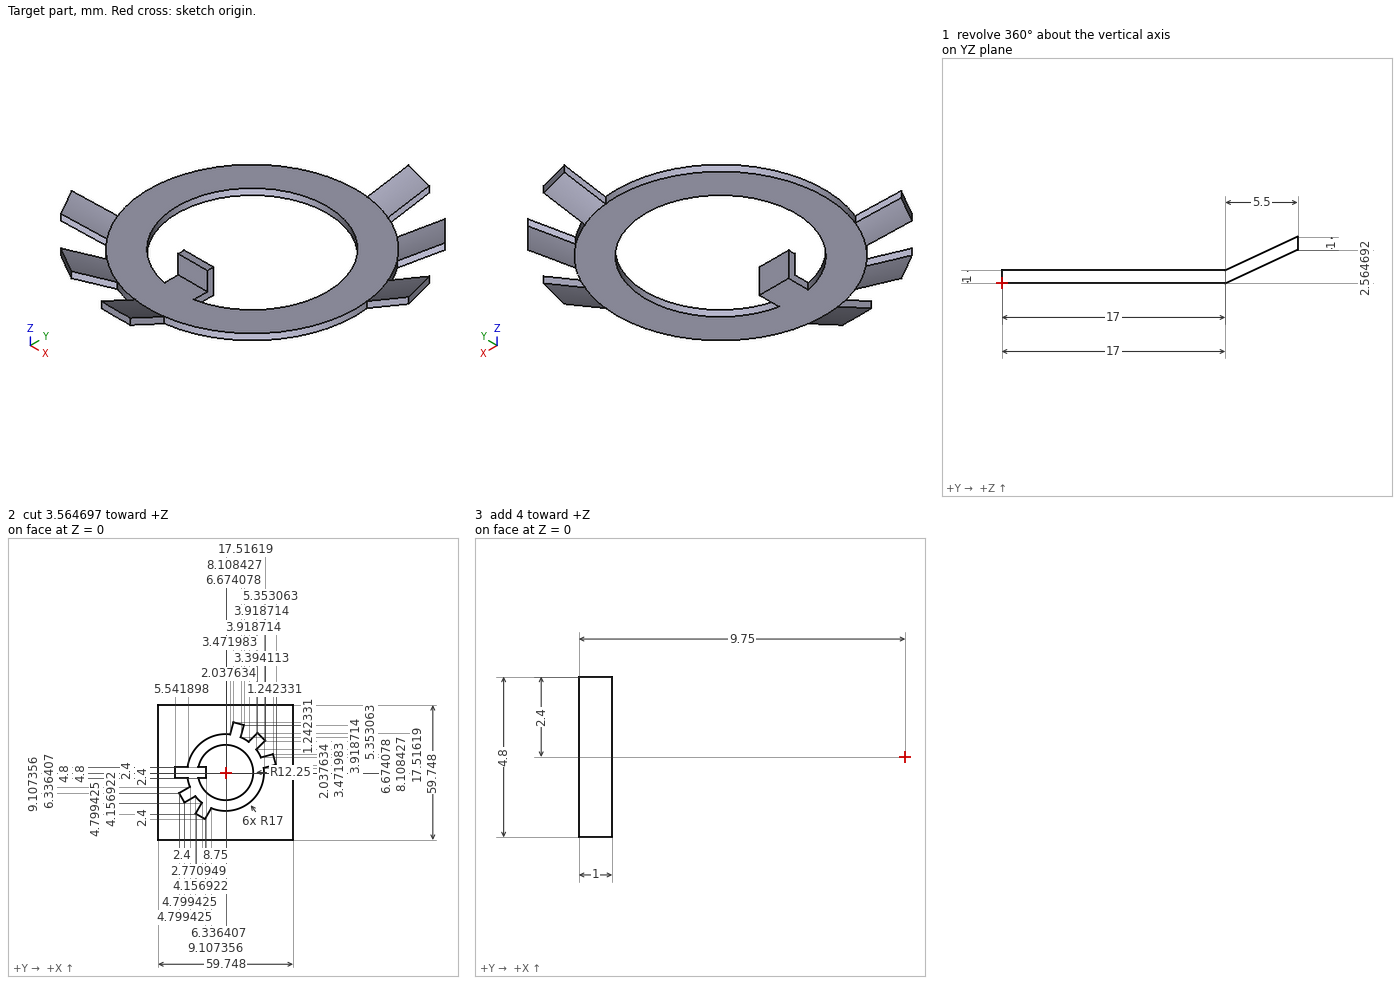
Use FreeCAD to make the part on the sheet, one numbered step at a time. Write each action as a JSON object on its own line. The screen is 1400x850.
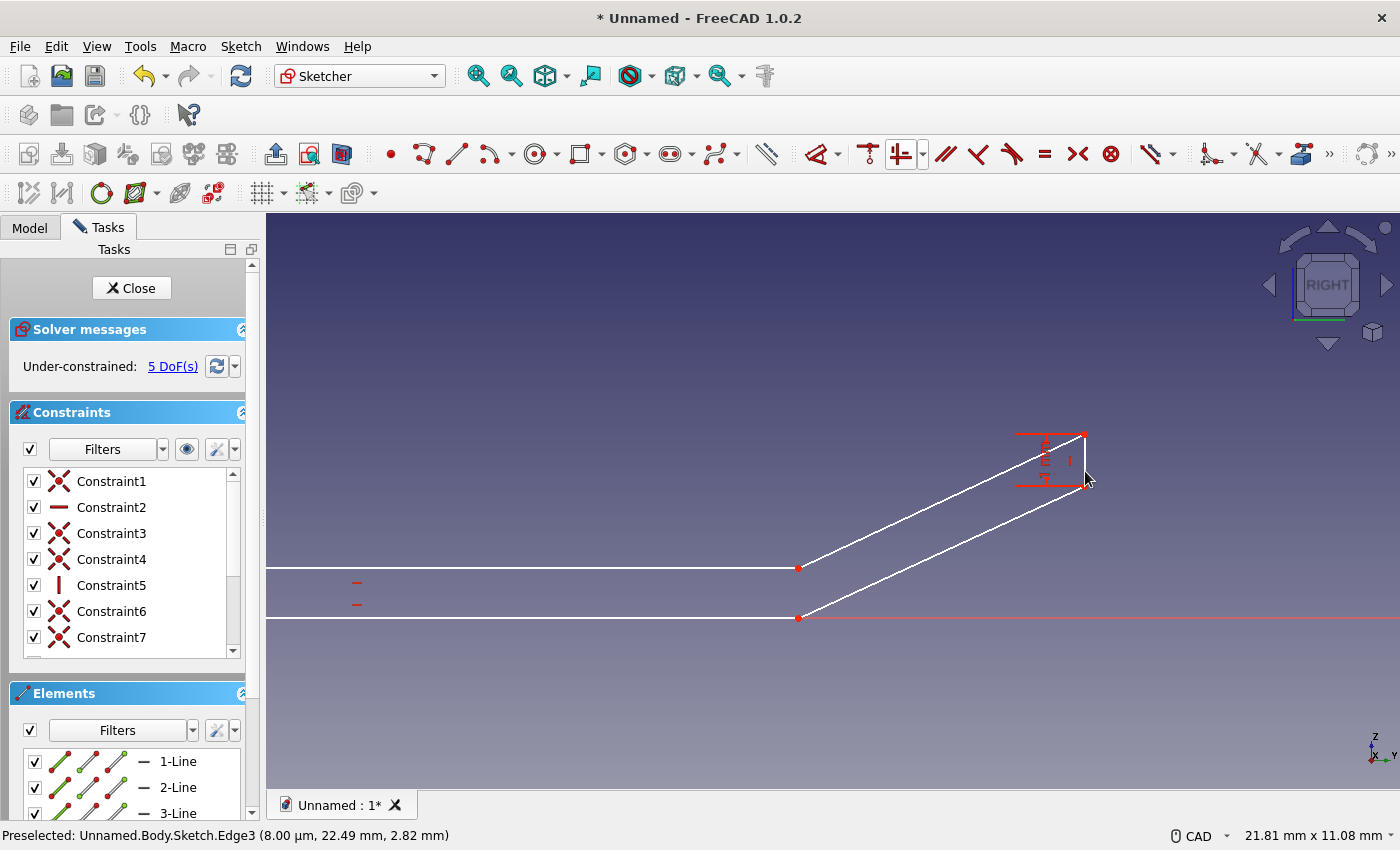
{"action": "scroll", "coordinate": [1086, 471], "scroll_direction": "down", "scroll_amount": 3}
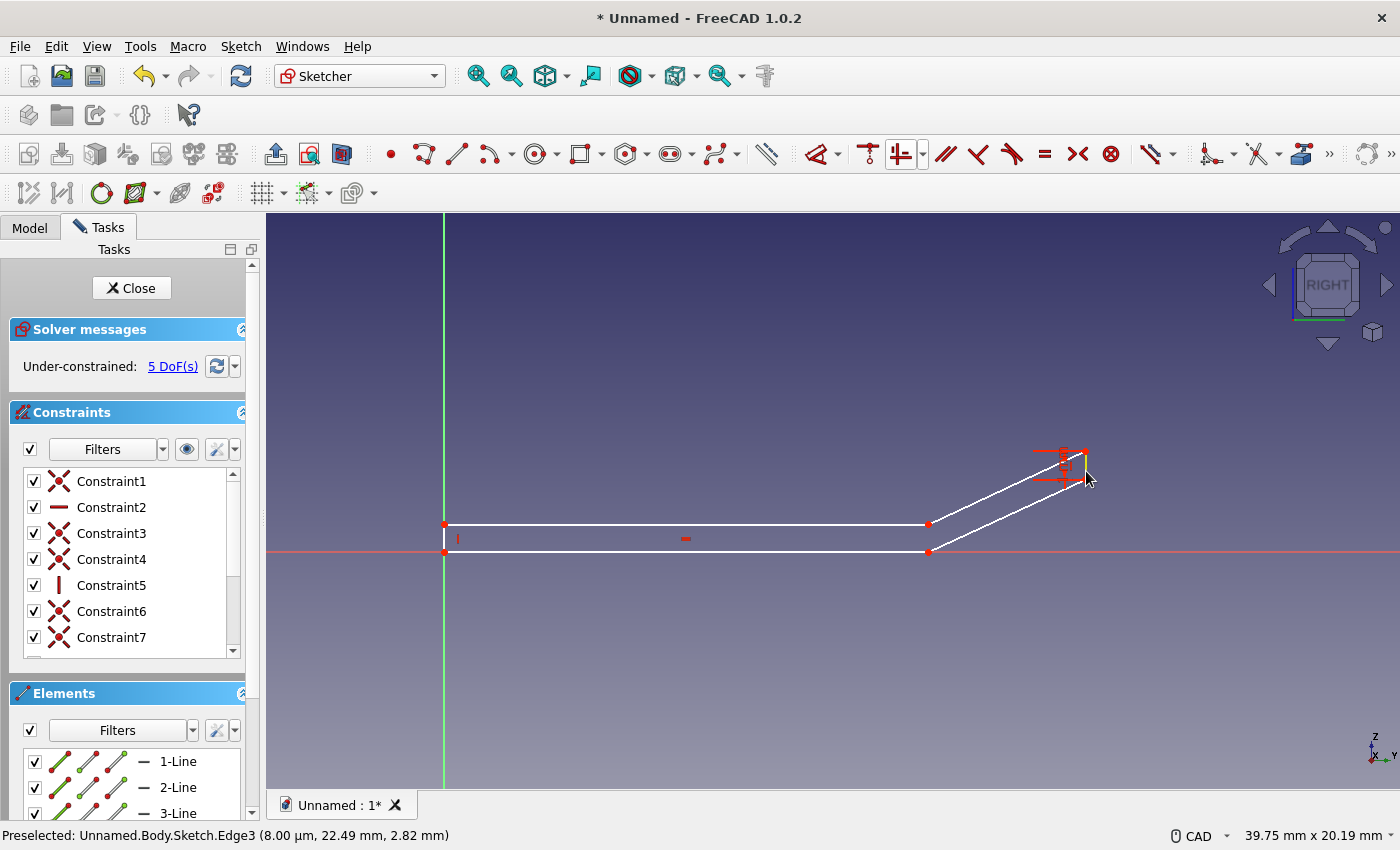
{"action": "scroll", "coordinate": [444, 533], "scroll_direction": "up", "scroll_amount": 3}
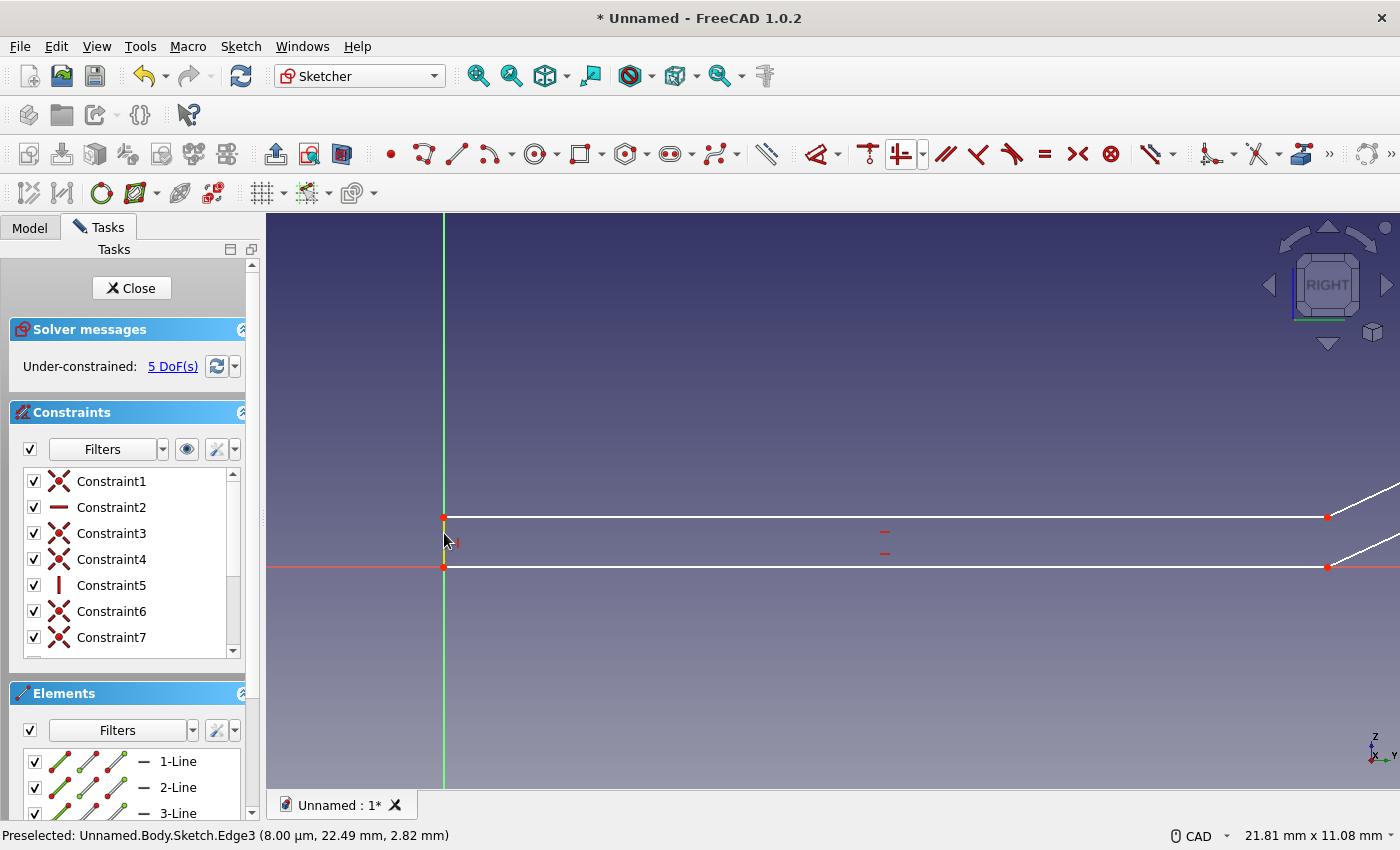
{"action": "left_click", "coordinate": [444, 532]}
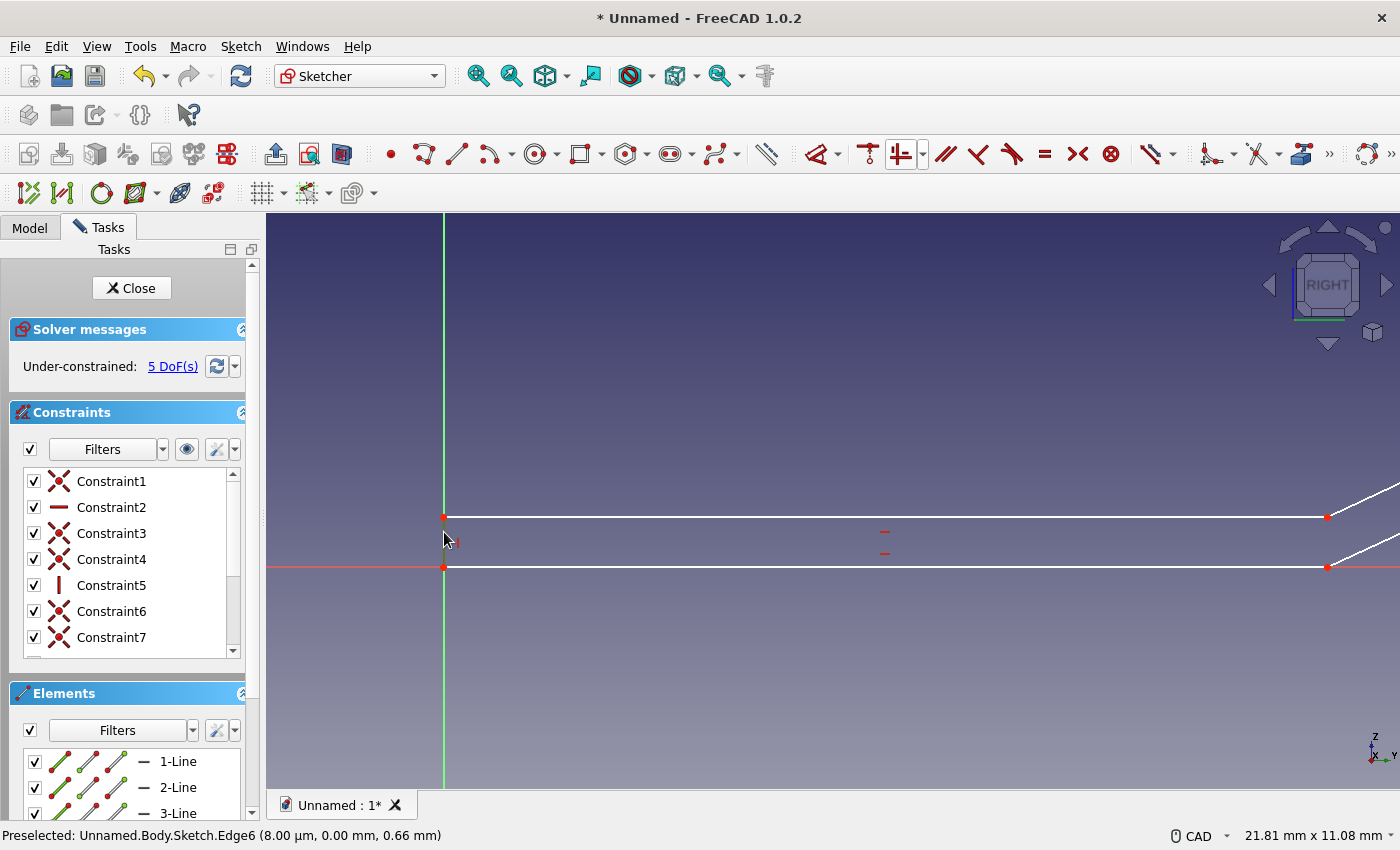
{"action": "key", "text": "i"}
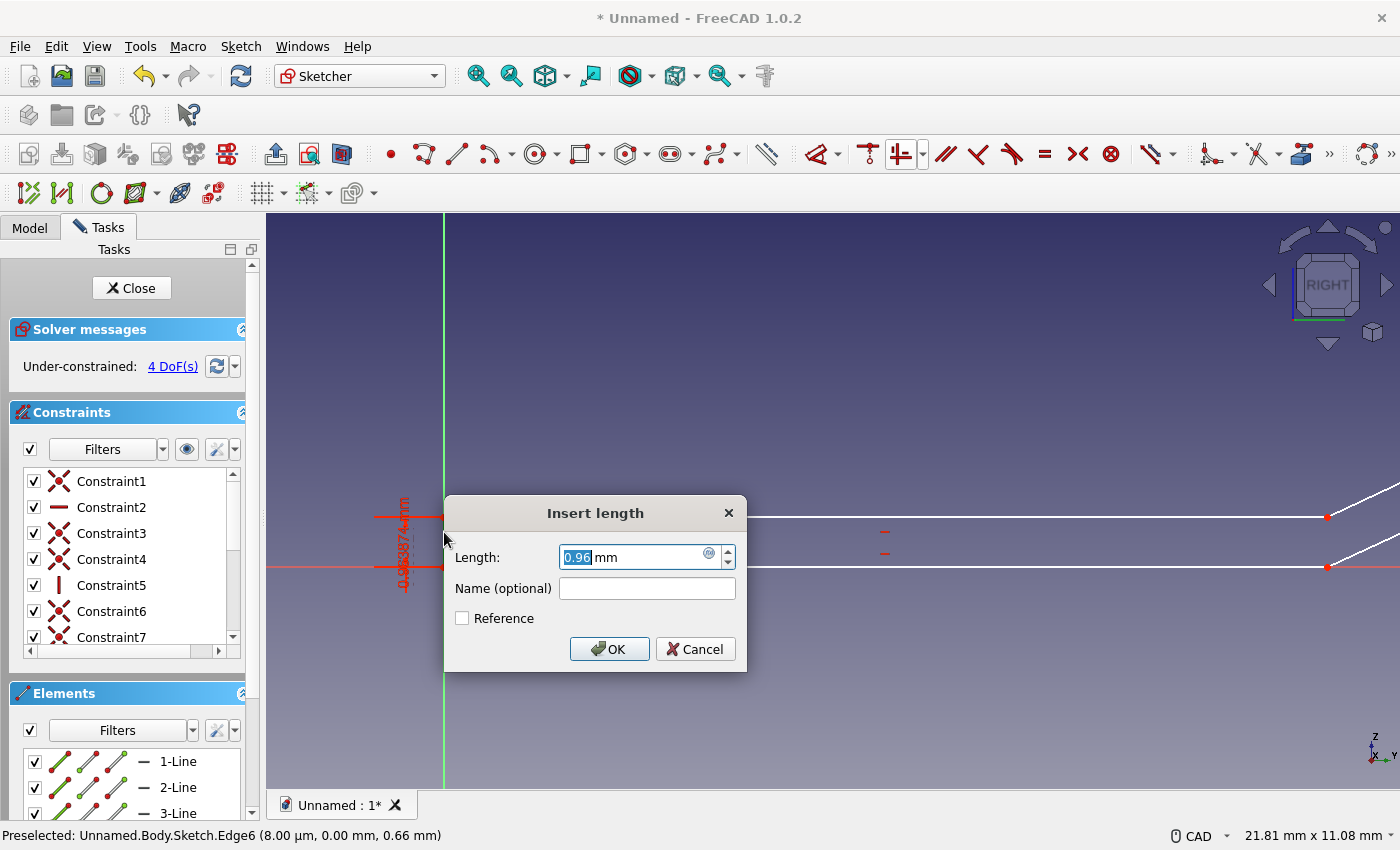
{"action": "type", "text": "1"}
{"action": "key", "text": "Return"}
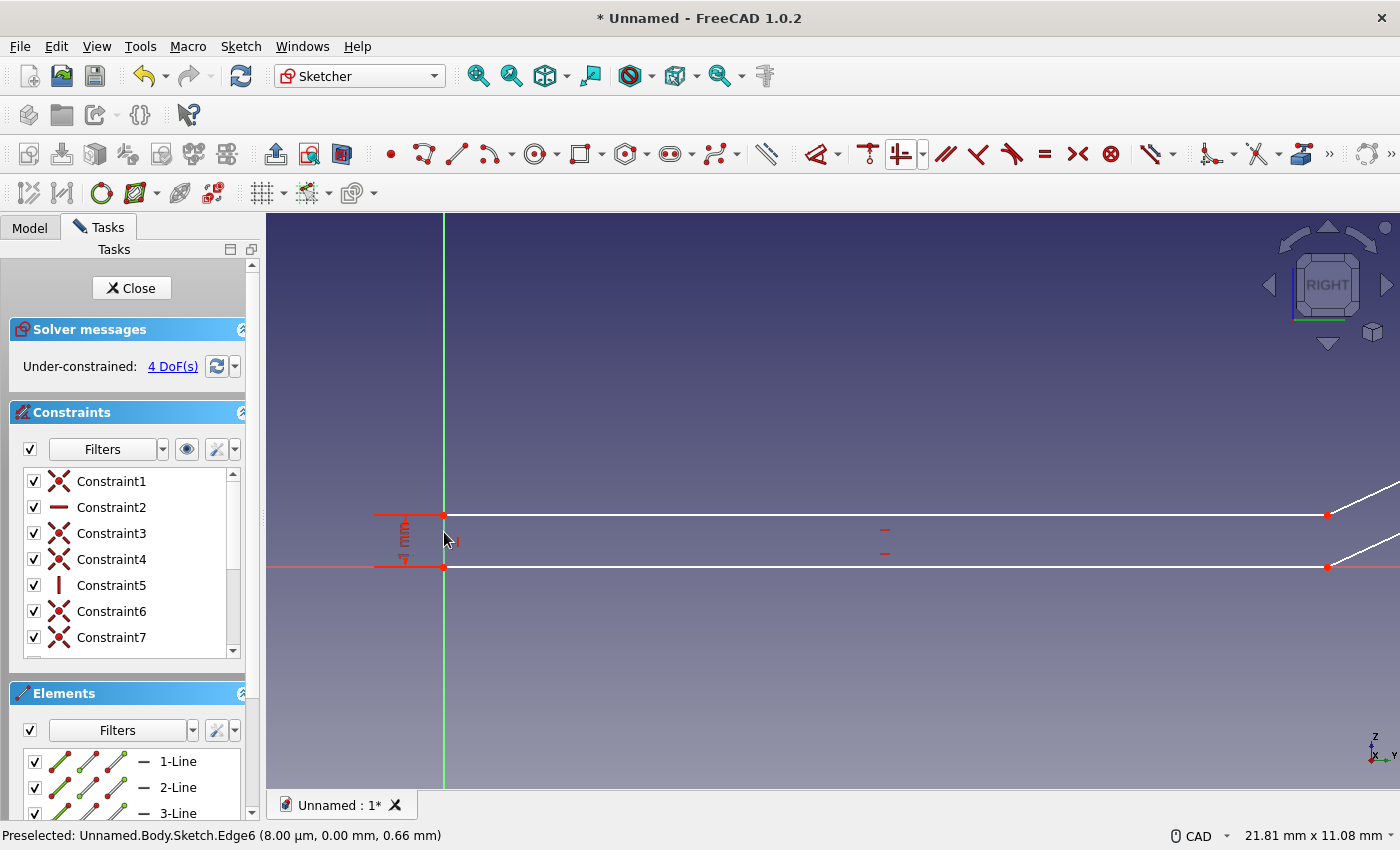
{"action": "left_click", "coordinate": [709, 567]}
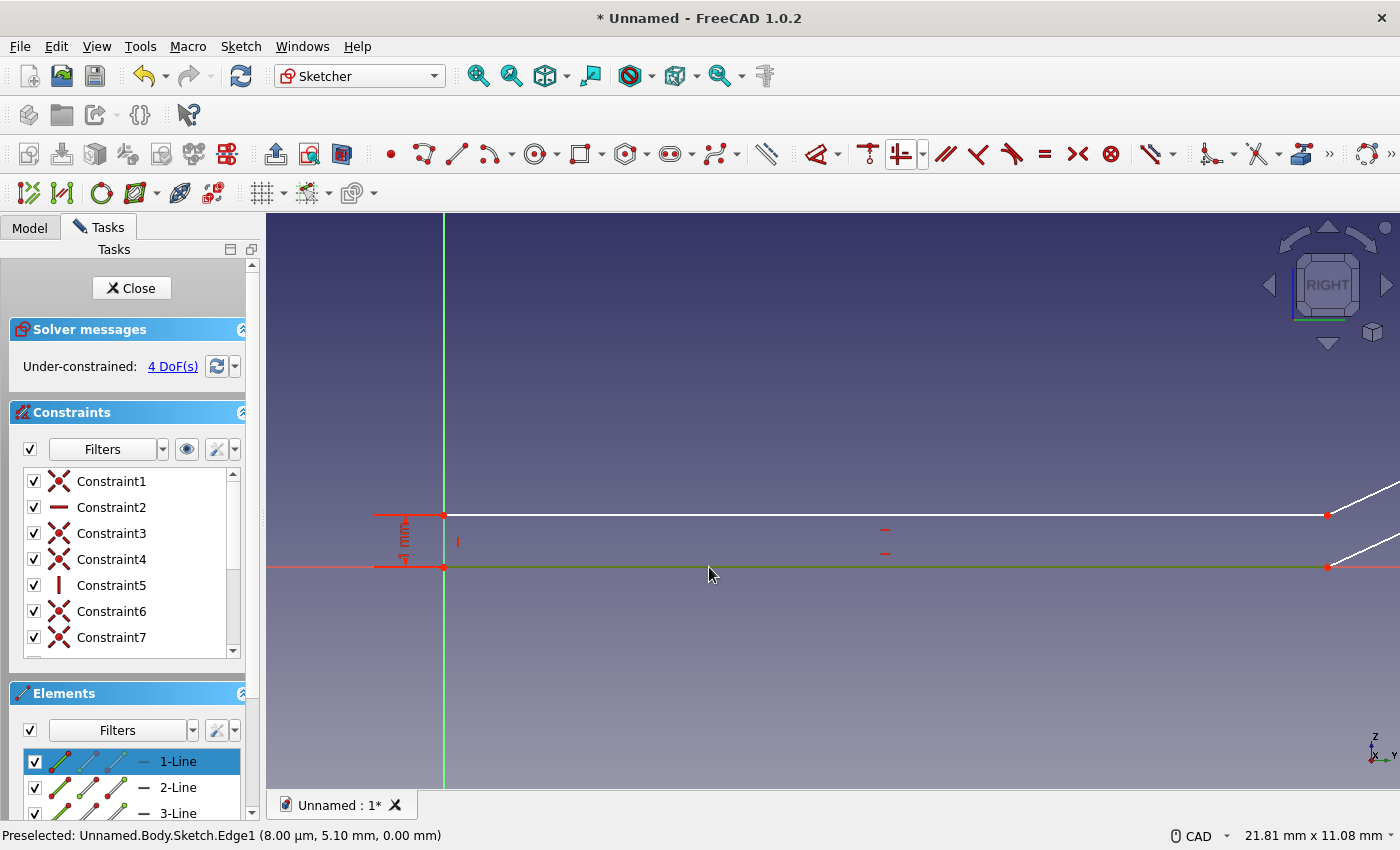
{"action": "key", "text": "l"}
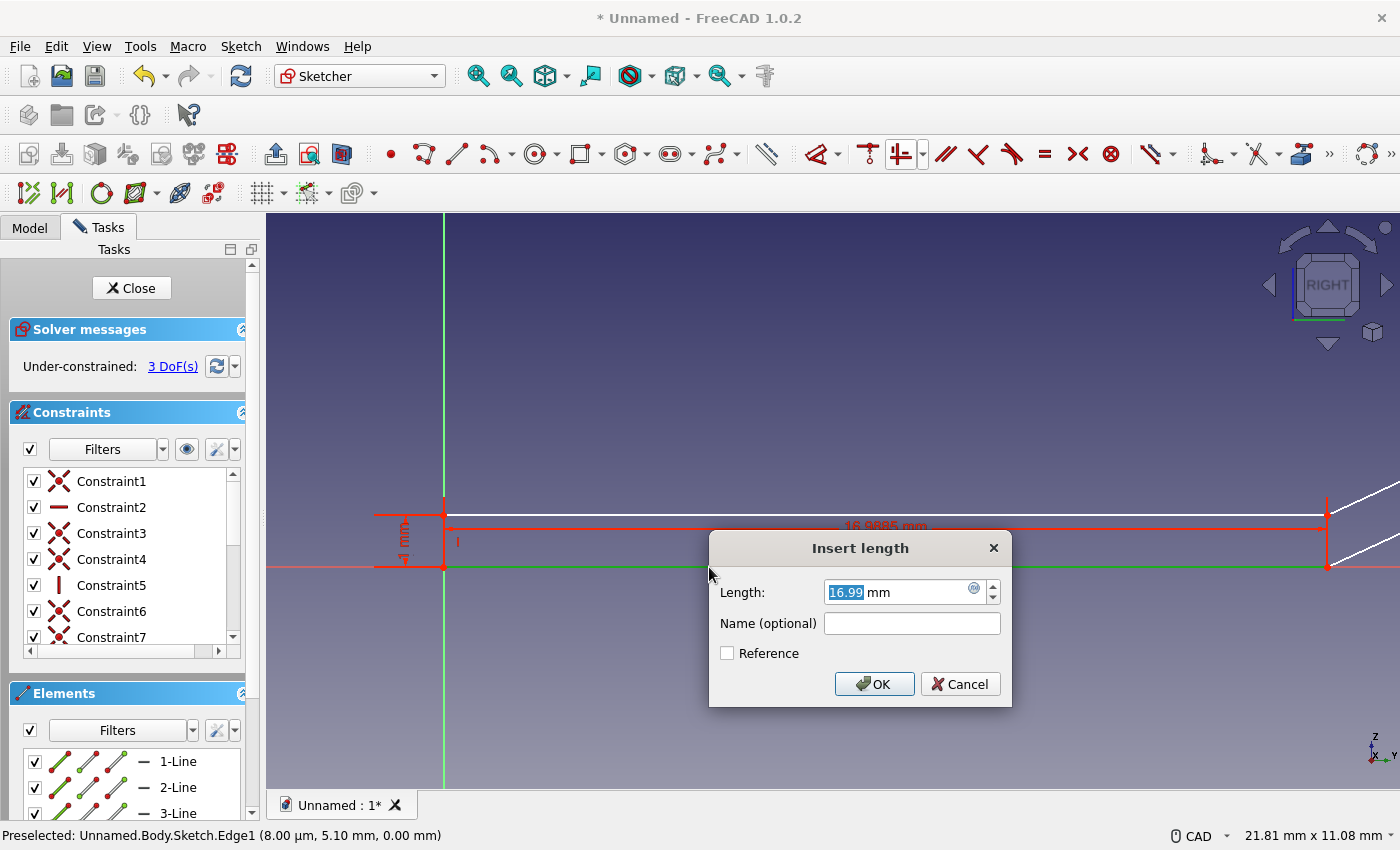
{"action": "type", "text": "17"}
{"action": "key", "text": "Return"}